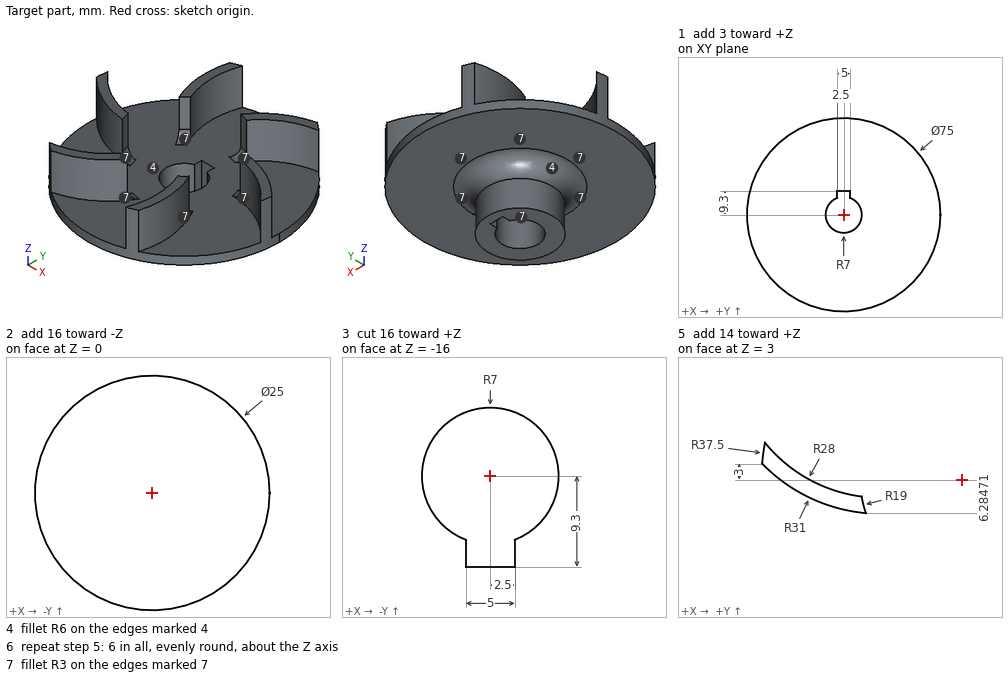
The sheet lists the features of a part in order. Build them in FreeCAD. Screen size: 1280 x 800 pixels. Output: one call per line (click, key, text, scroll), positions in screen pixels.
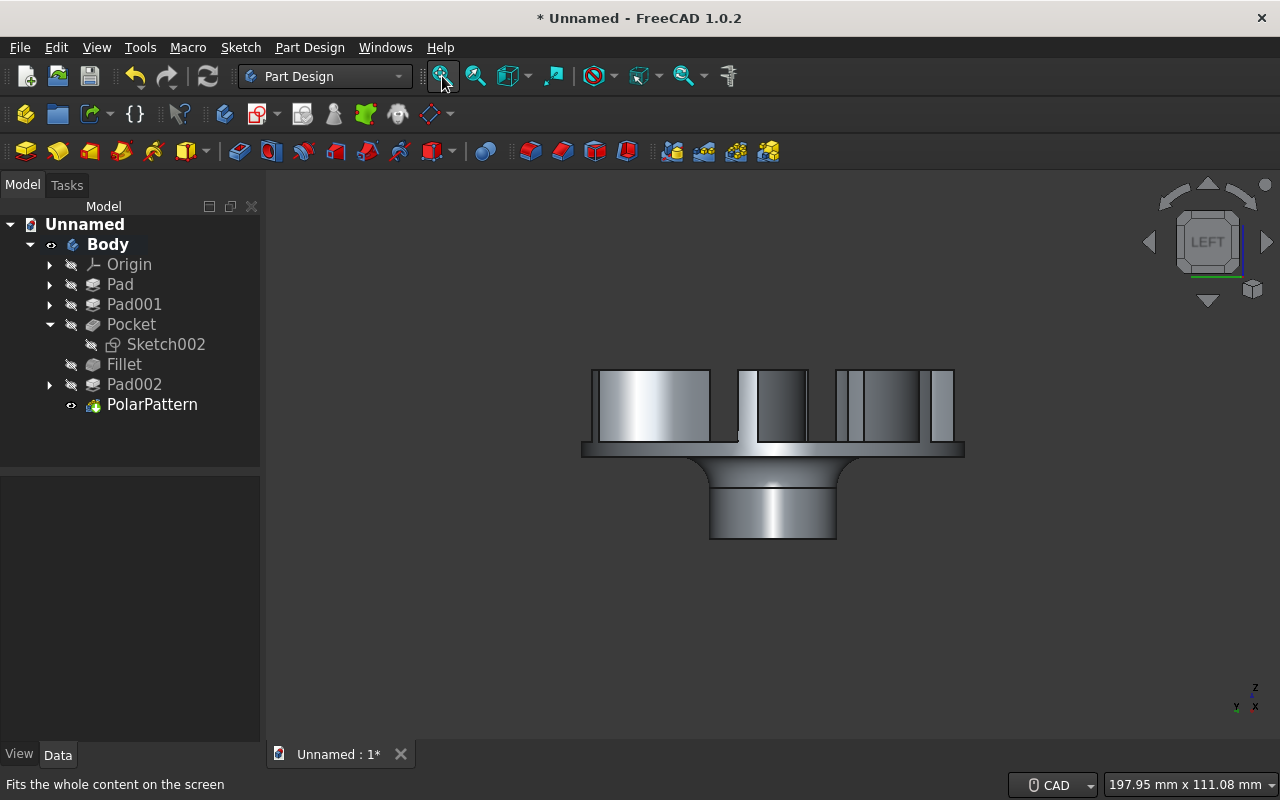
scroll(704, 441, up, 5)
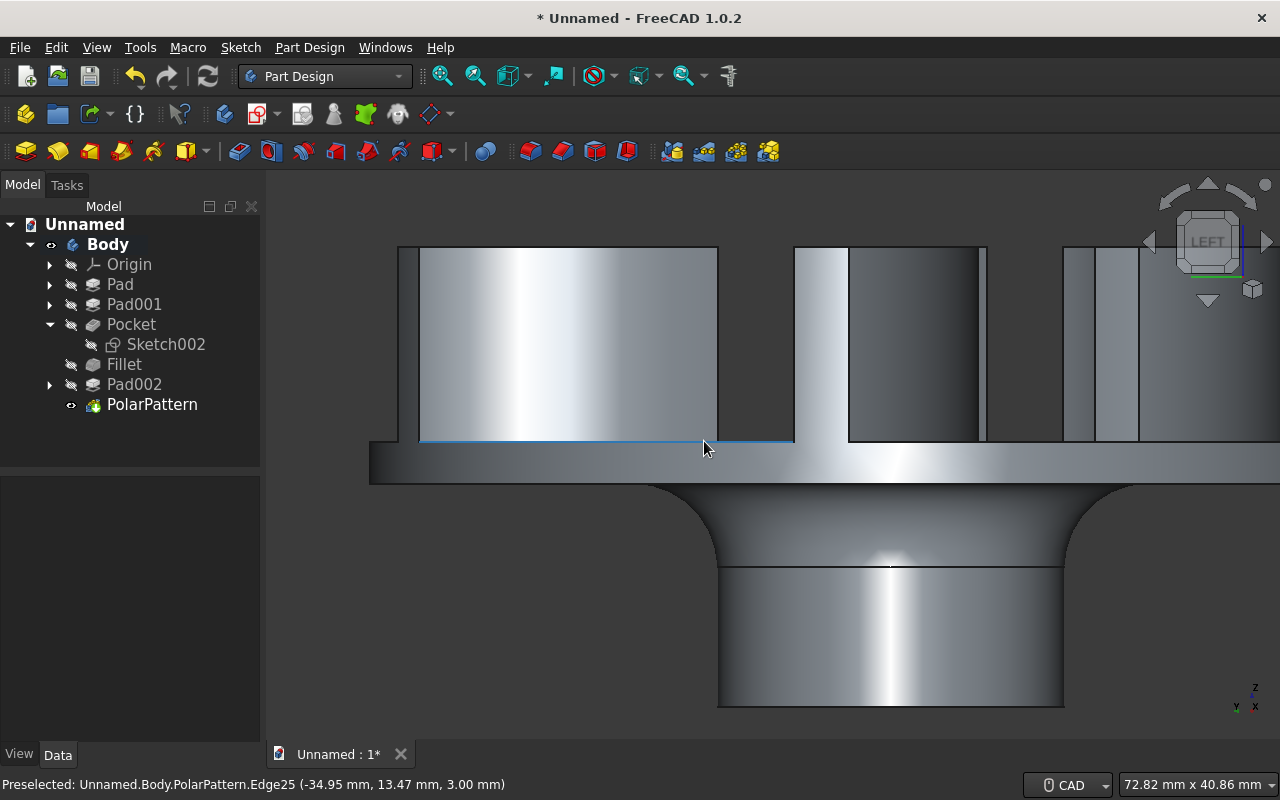
key(v)
key(f)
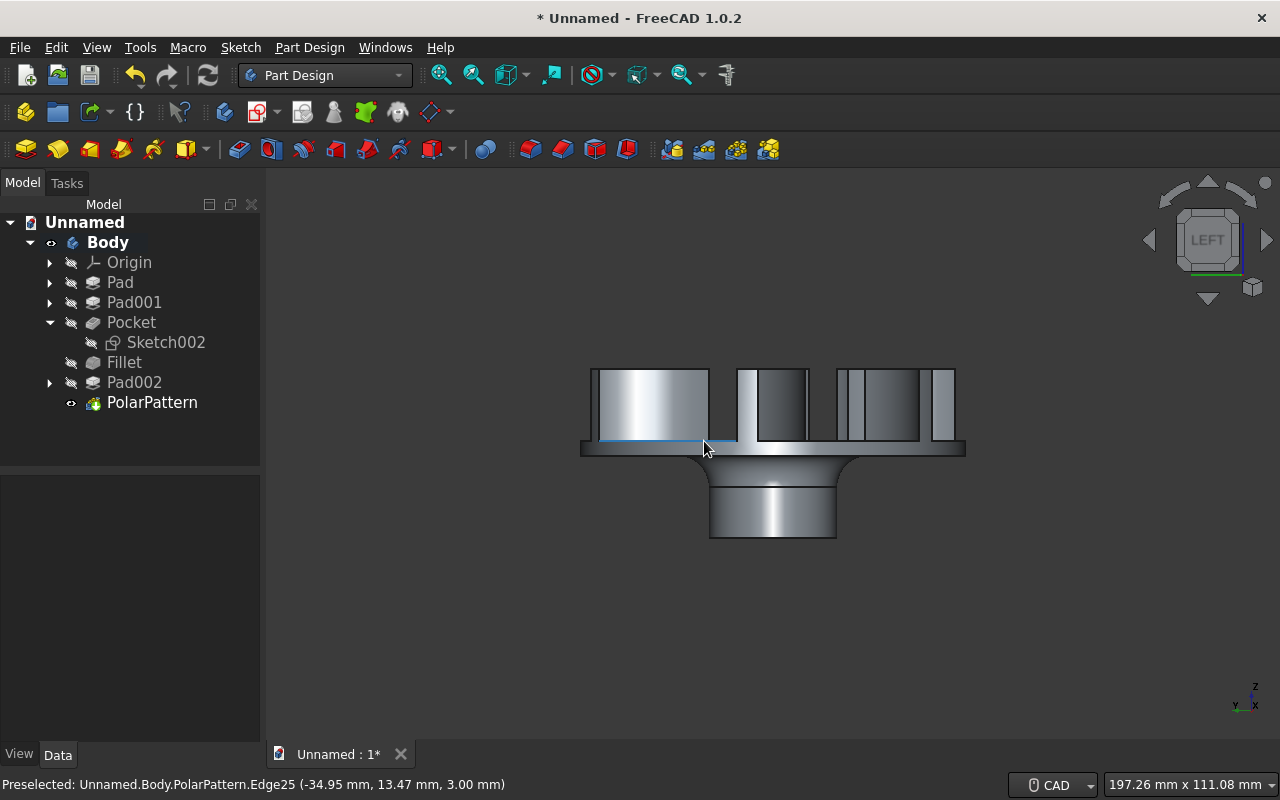
key(v)
key(3)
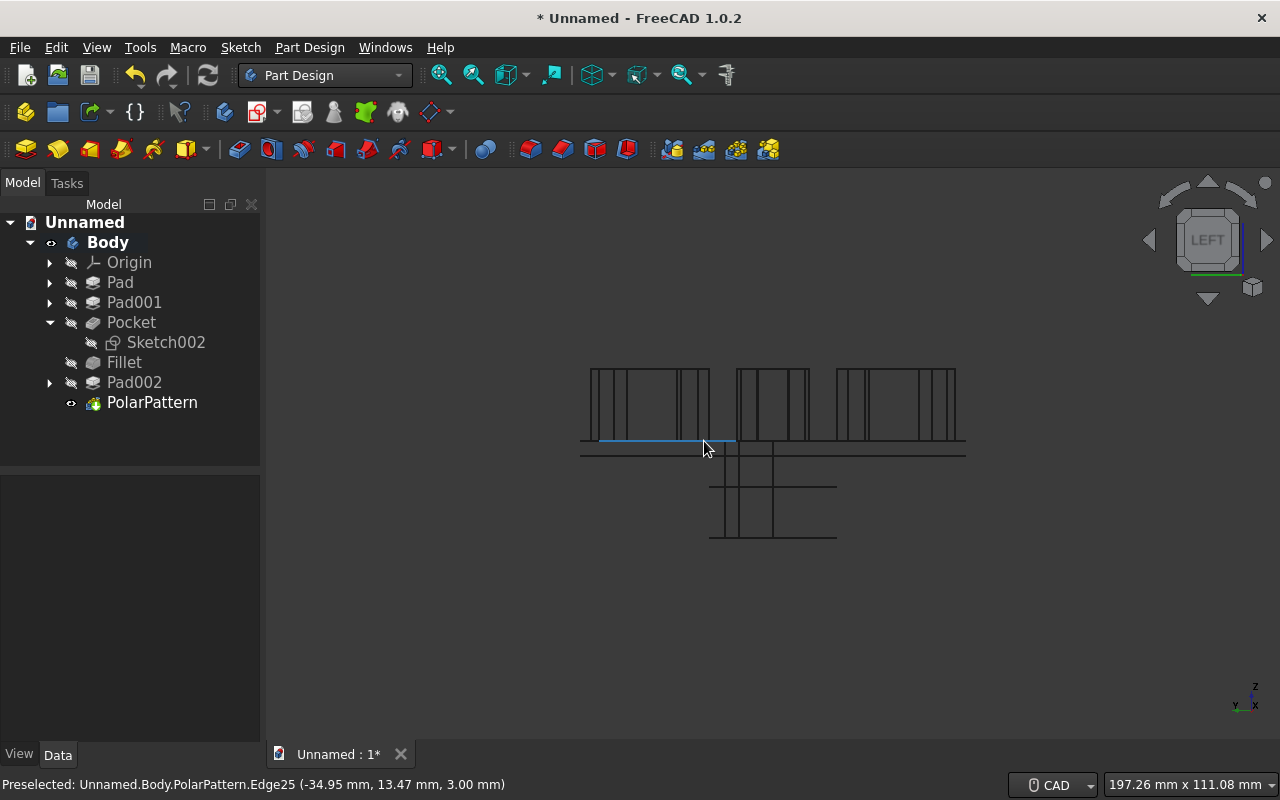
key(0)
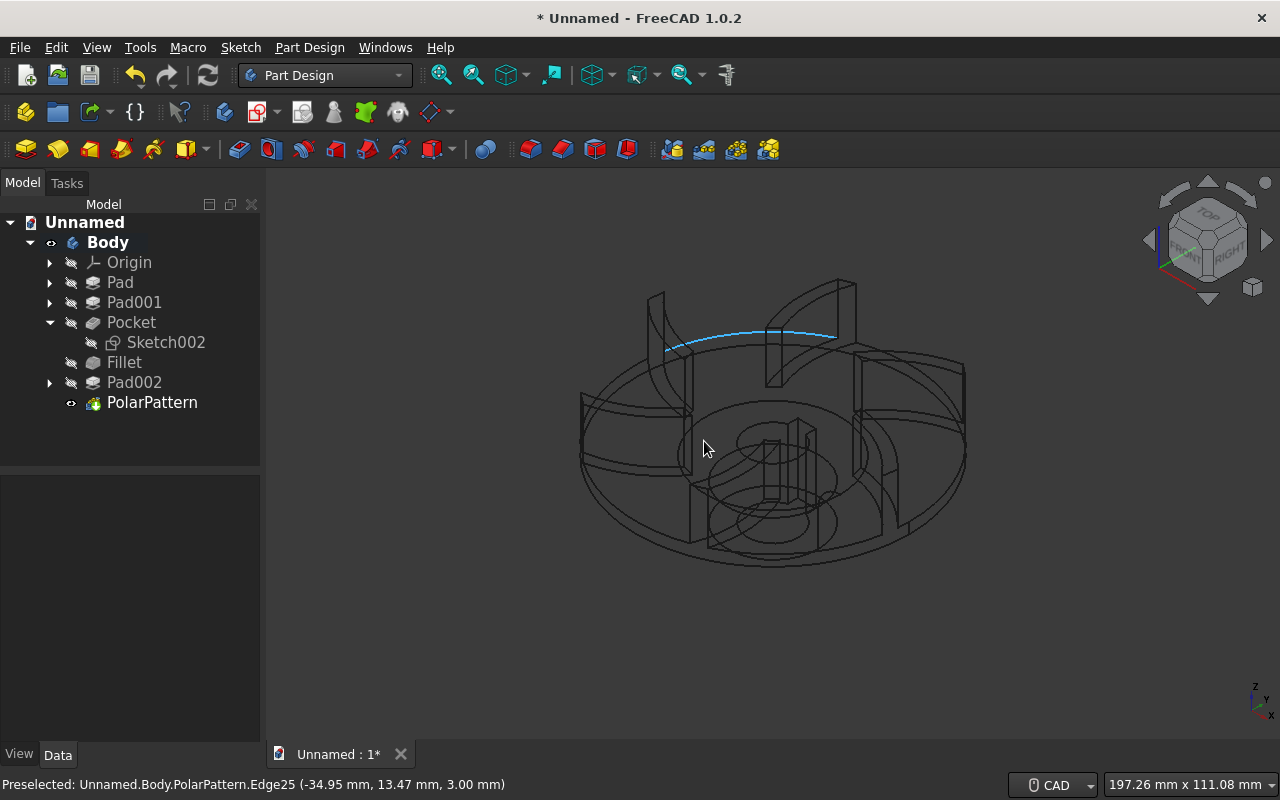
click(774, 386)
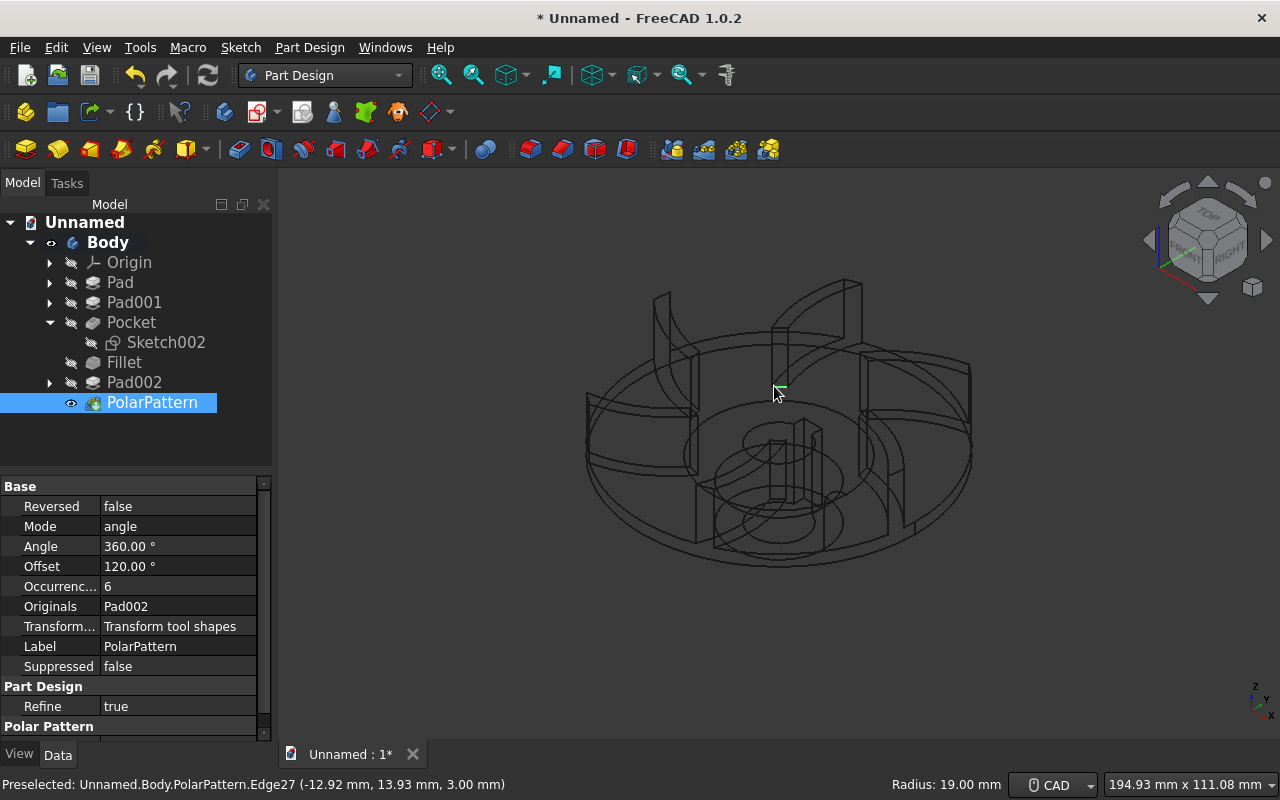
click(692, 468, ctrl)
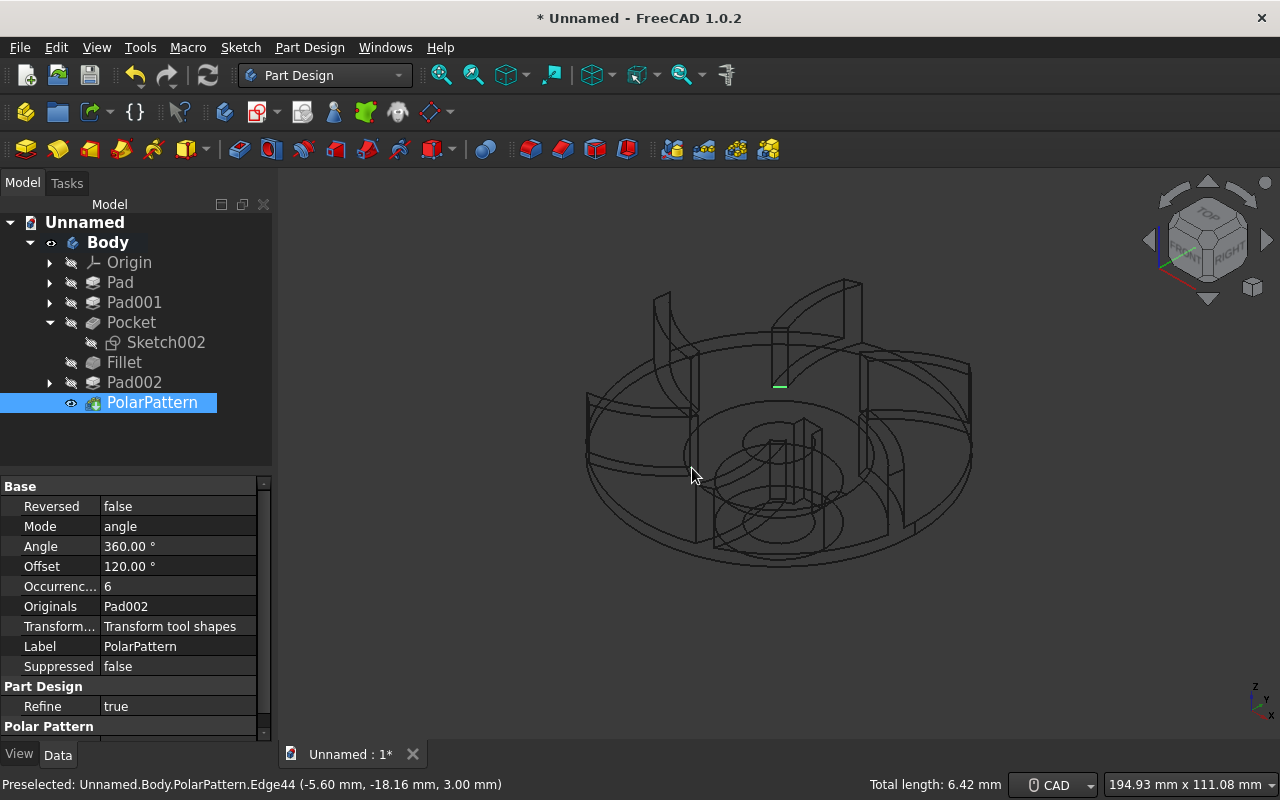
click(778, 498, ctrl)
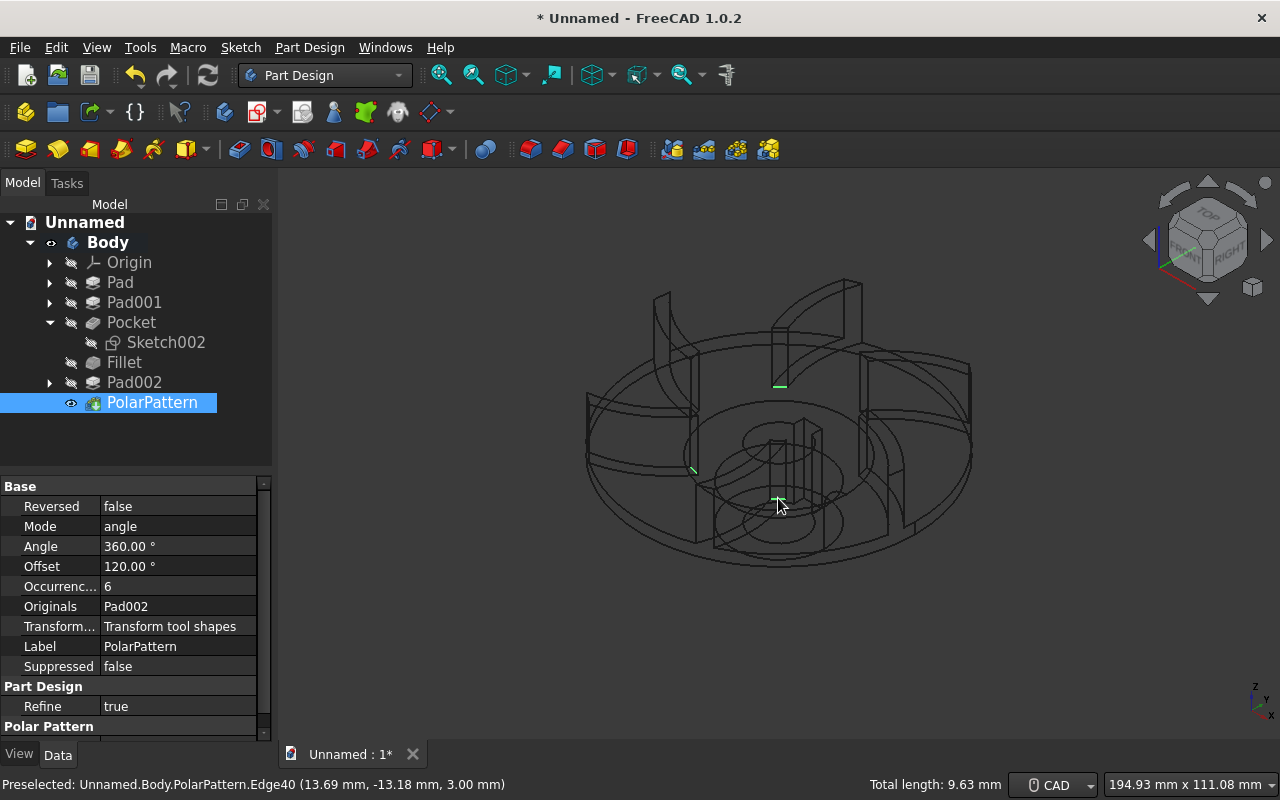
click(865, 469, ctrl)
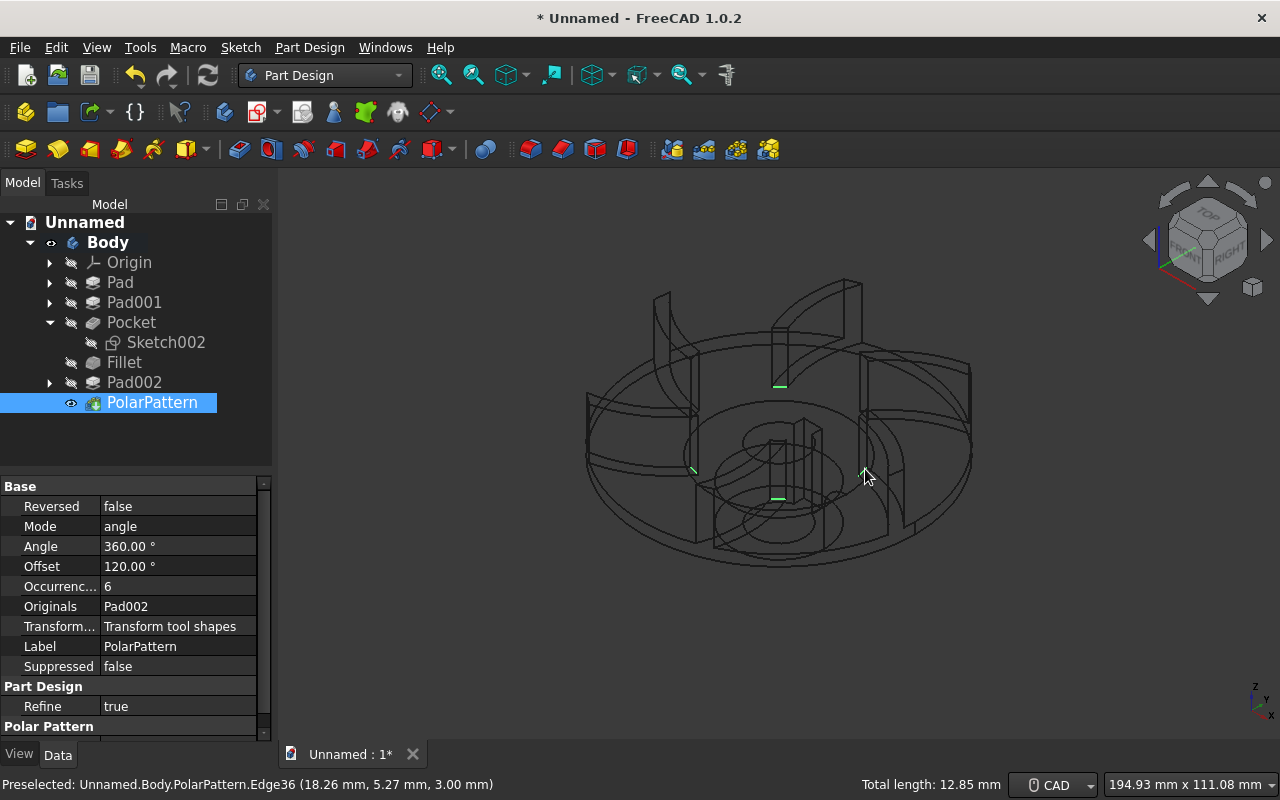
scroll(695, 413, up, 5)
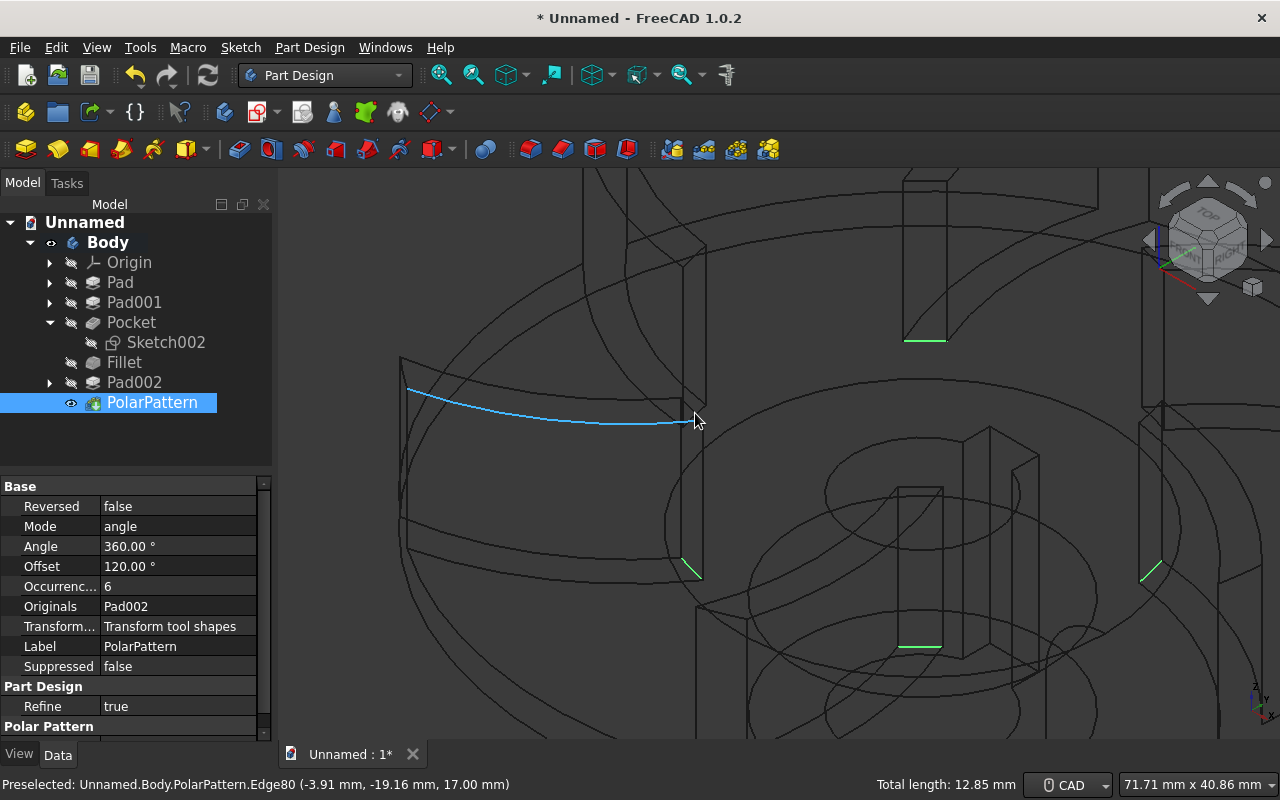
click(701, 408, ctrl)